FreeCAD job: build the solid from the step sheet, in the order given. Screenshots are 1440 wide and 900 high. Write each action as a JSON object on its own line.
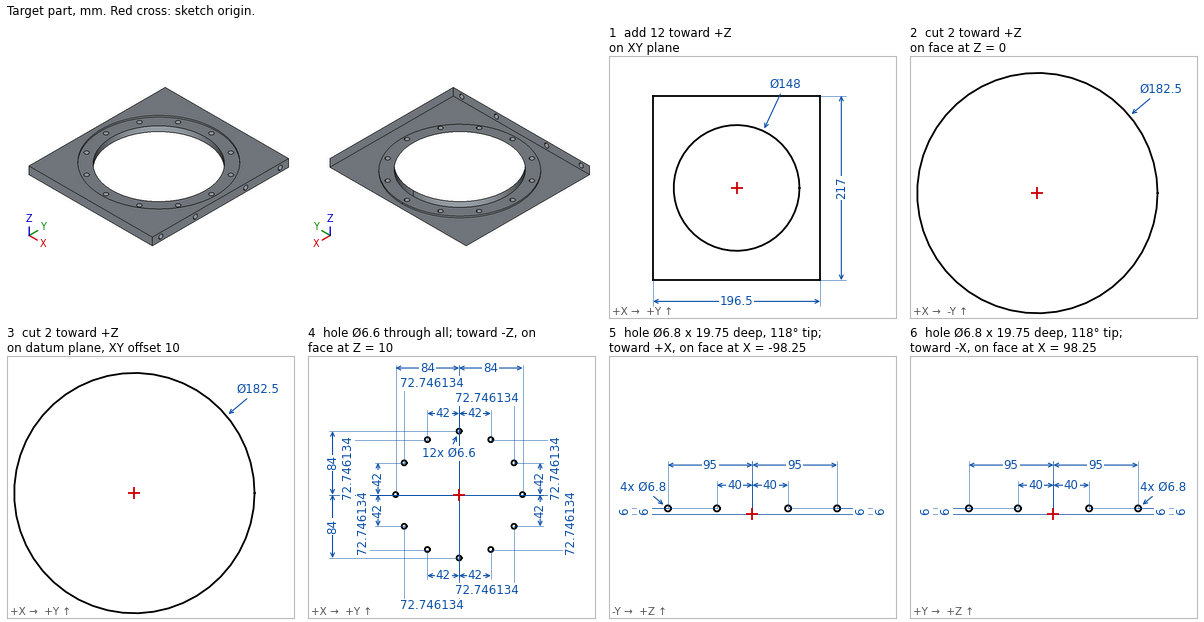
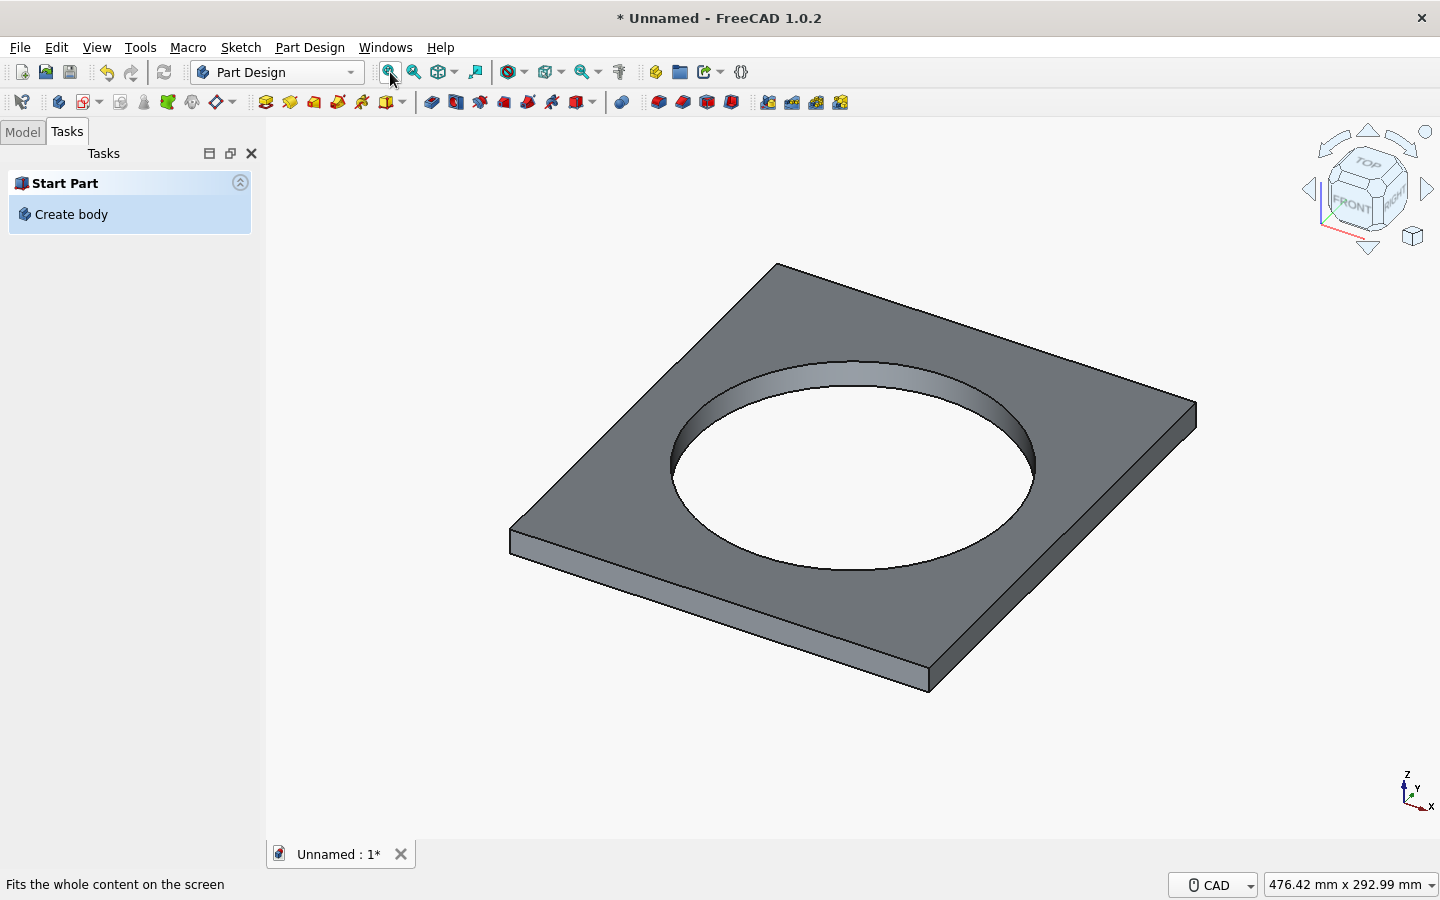
{"action": "key", "text": "5"}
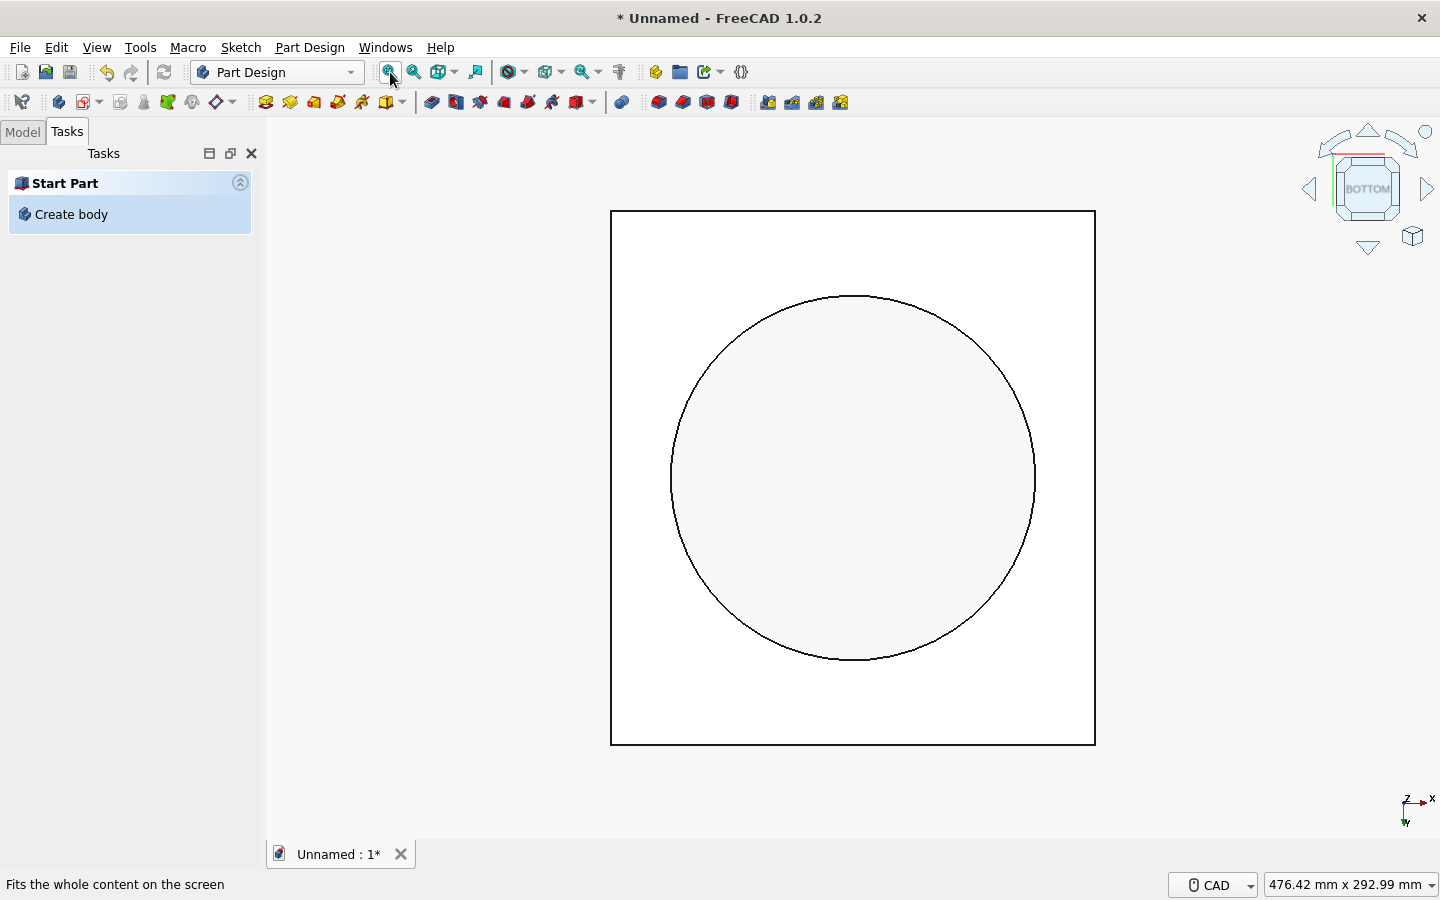
{"action": "left_click", "coordinate": [991, 706]}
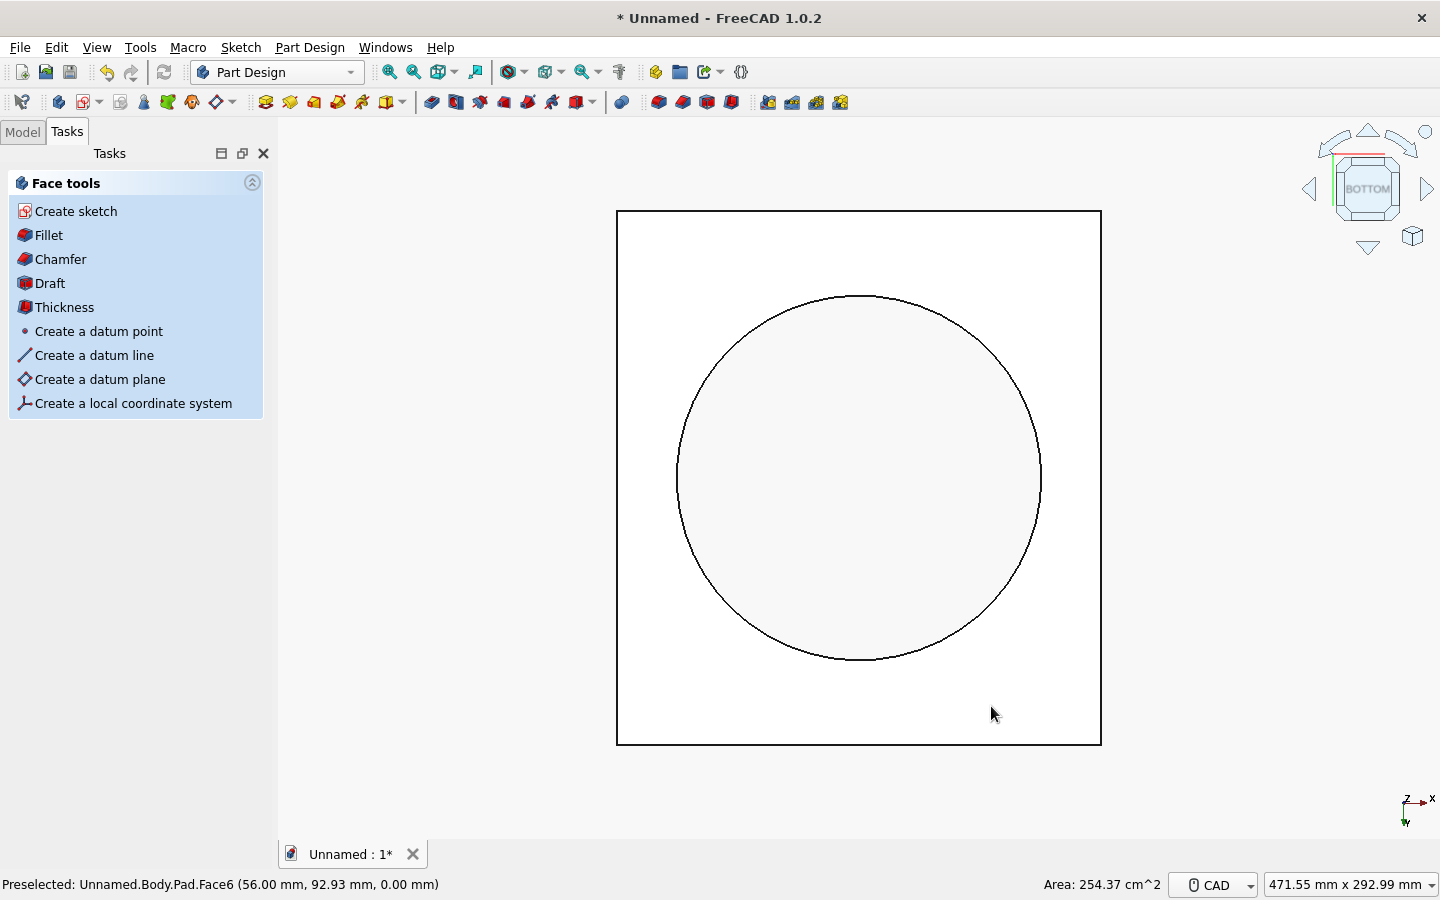
{"action": "left_click", "coordinate": [84, 102]}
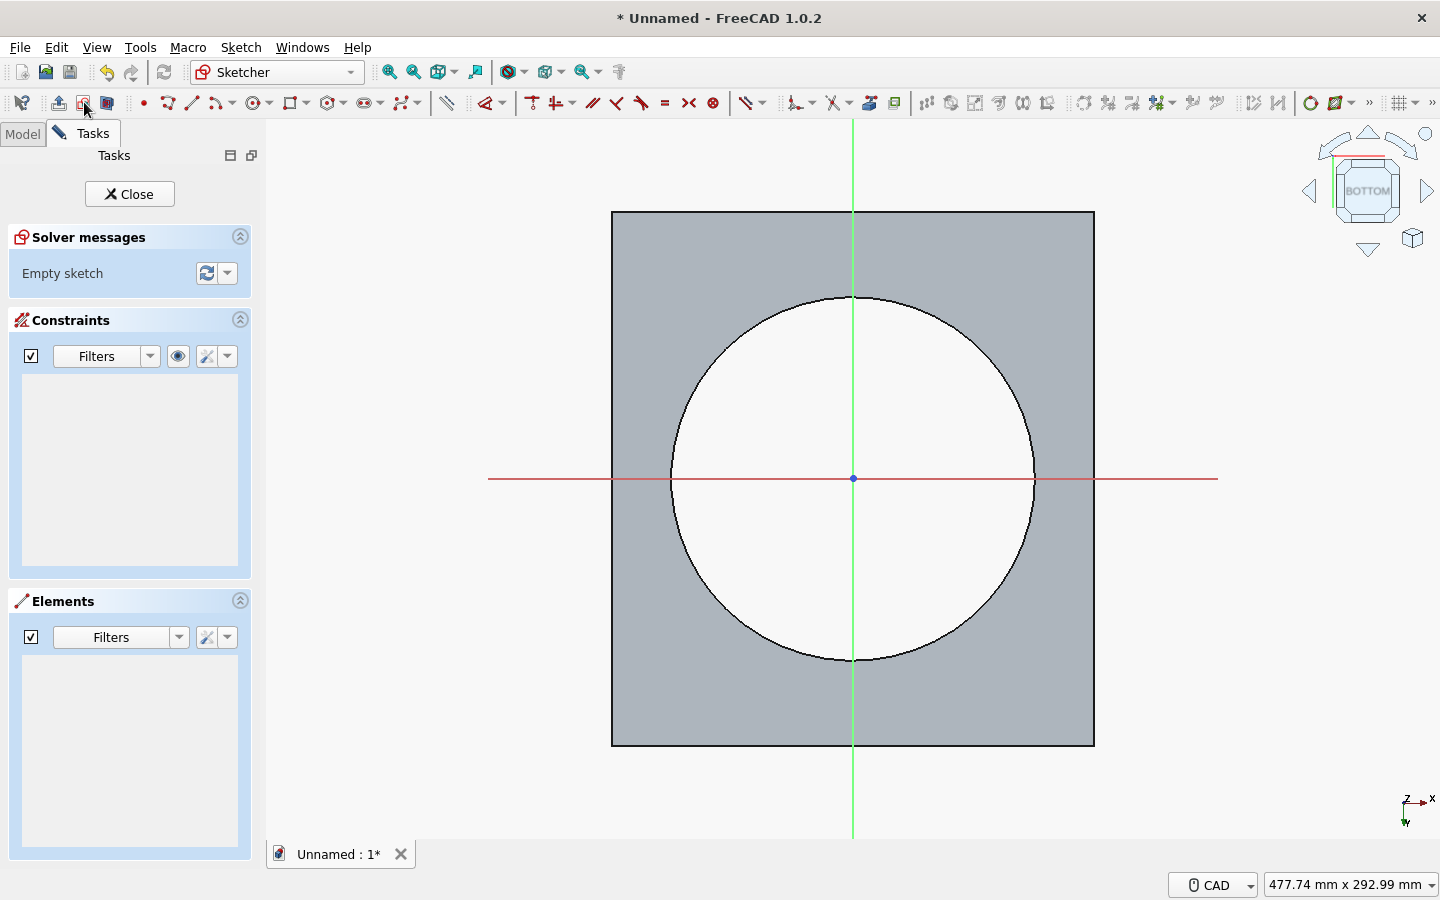
{"action": "left_click", "coordinate": [254, 104]}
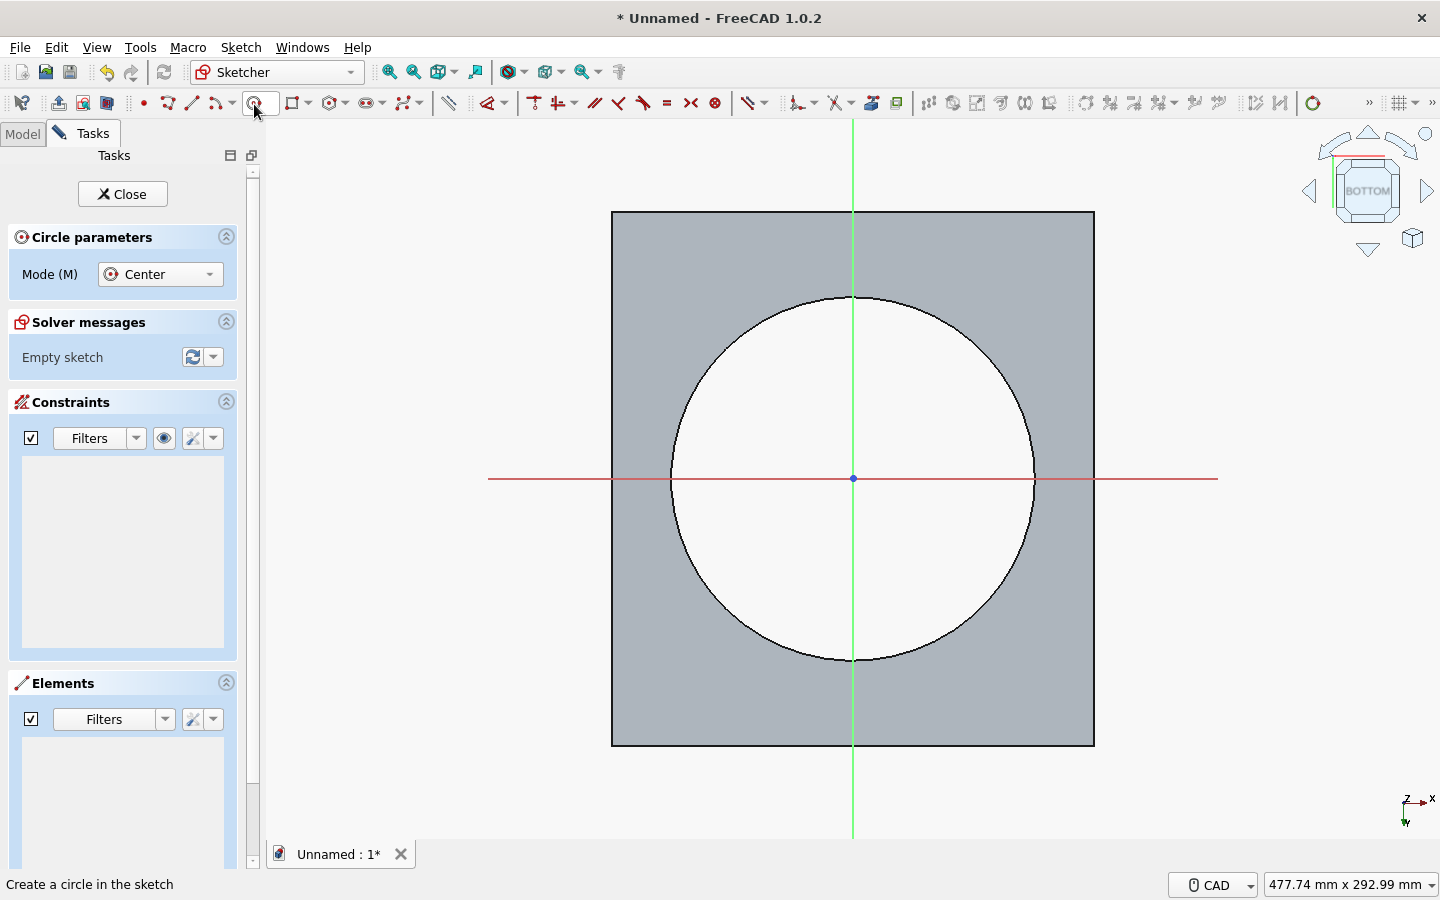
{"action": "left_click", "coordinate": [853, 479]}
{"action": "mouse_move", "coordinate": [1012, 320]}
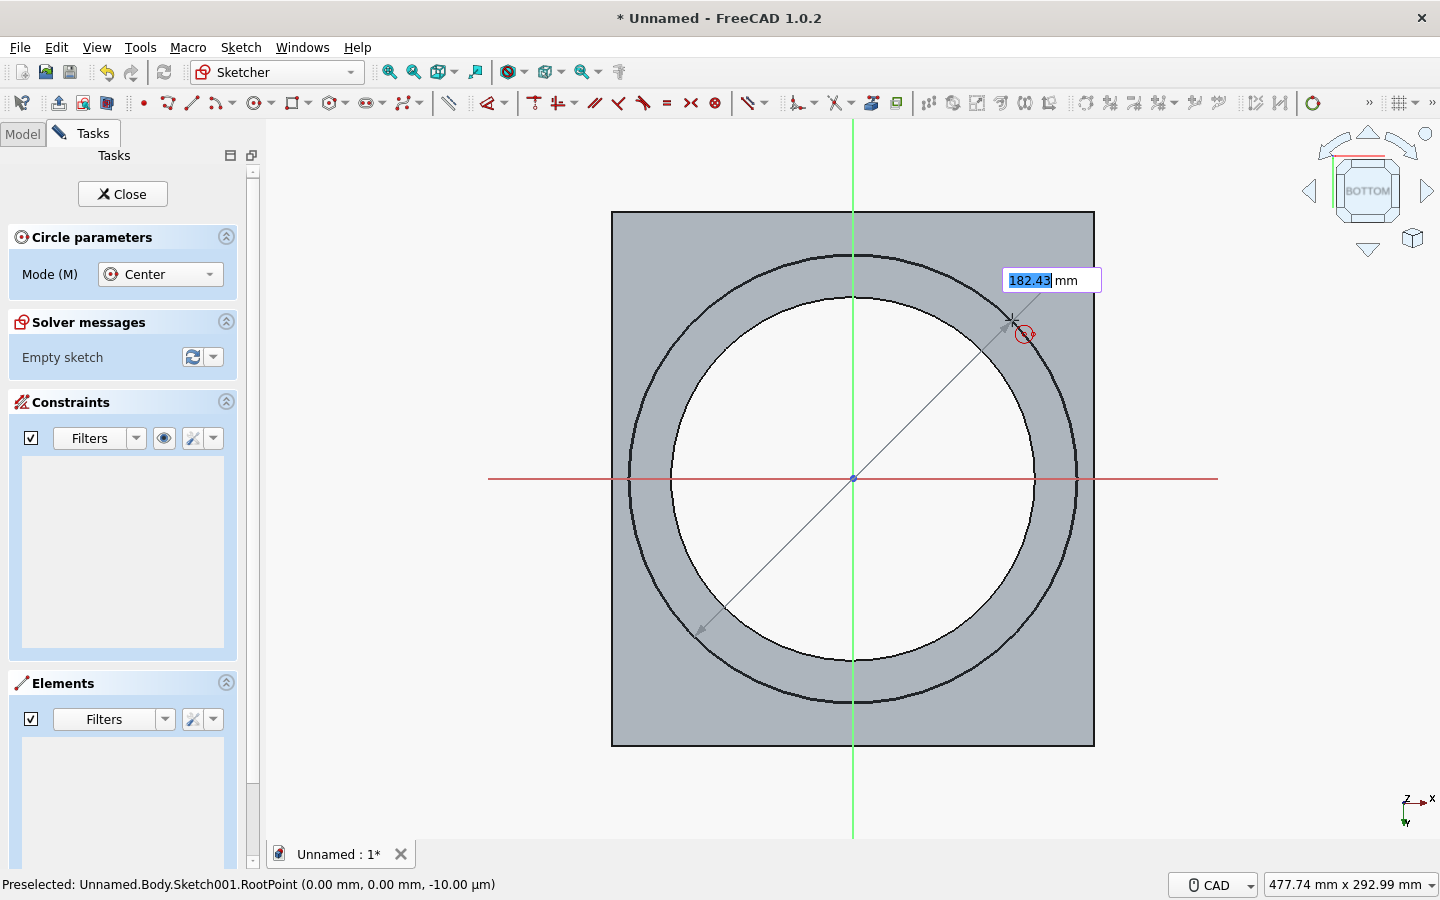
{"action": "type", "text": "182.5"}
{"action": "key", "text": "Return"}
{"action": "key", "text": "Escape"}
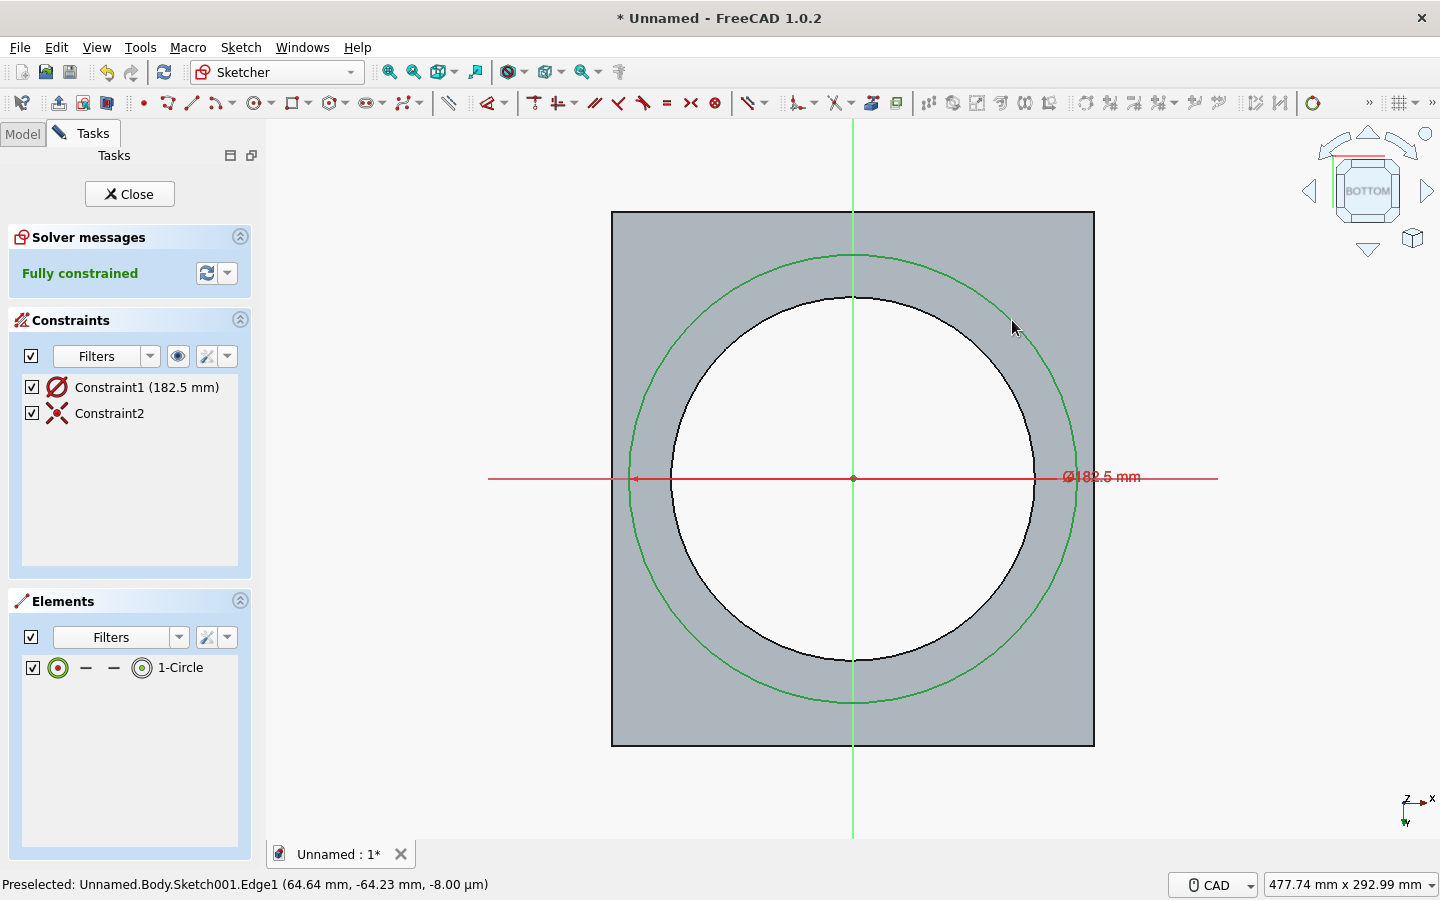
{"action": "left_click", "coordinate": [130, 194]}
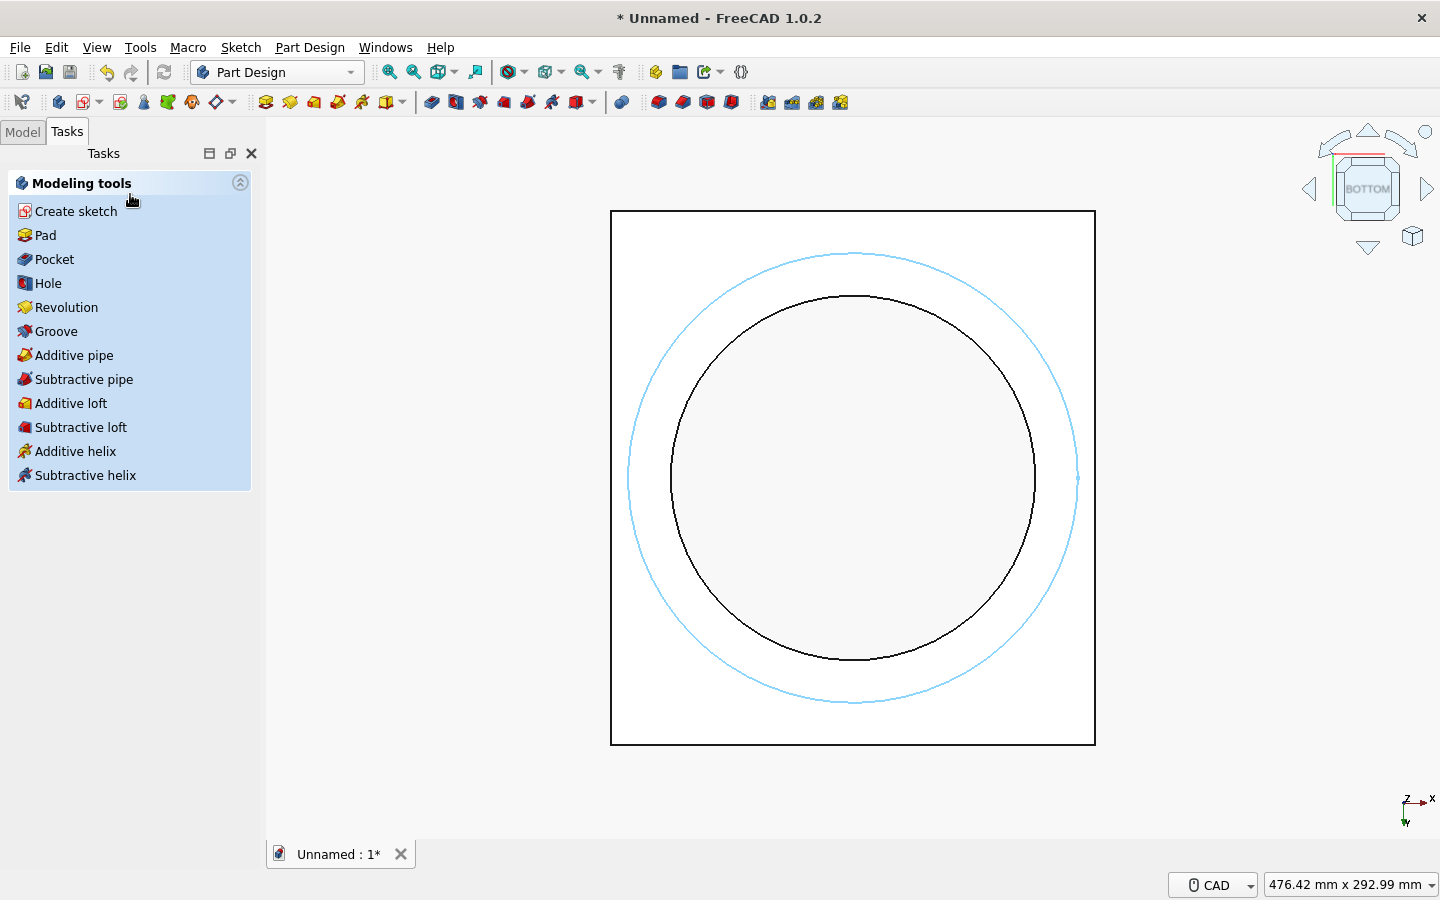
{"action": "left_click", "coordinate": [432, 102]}